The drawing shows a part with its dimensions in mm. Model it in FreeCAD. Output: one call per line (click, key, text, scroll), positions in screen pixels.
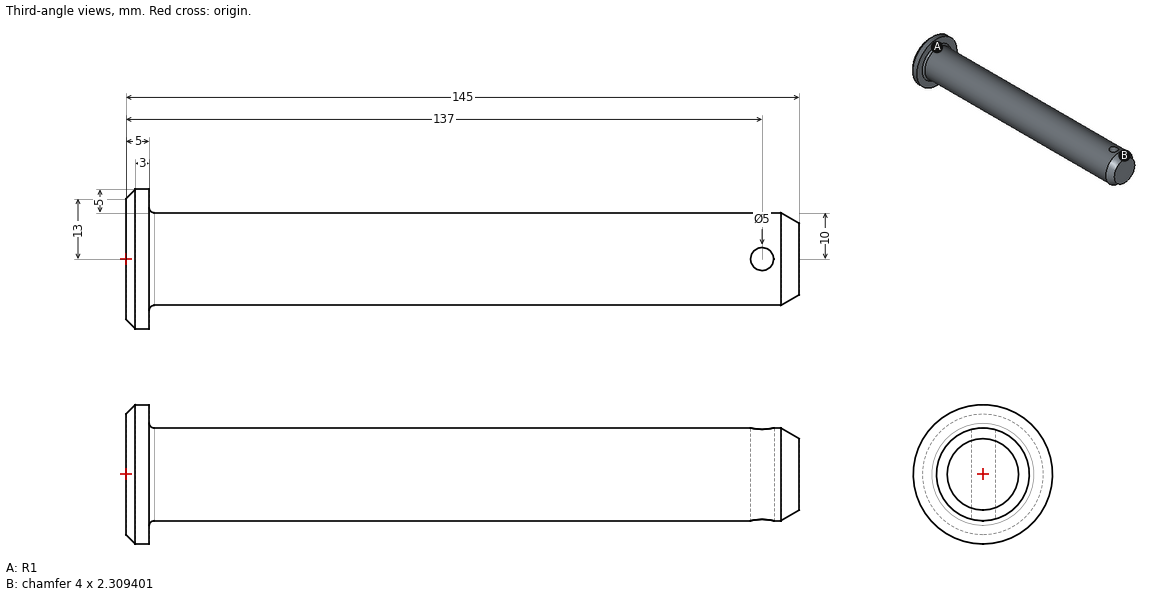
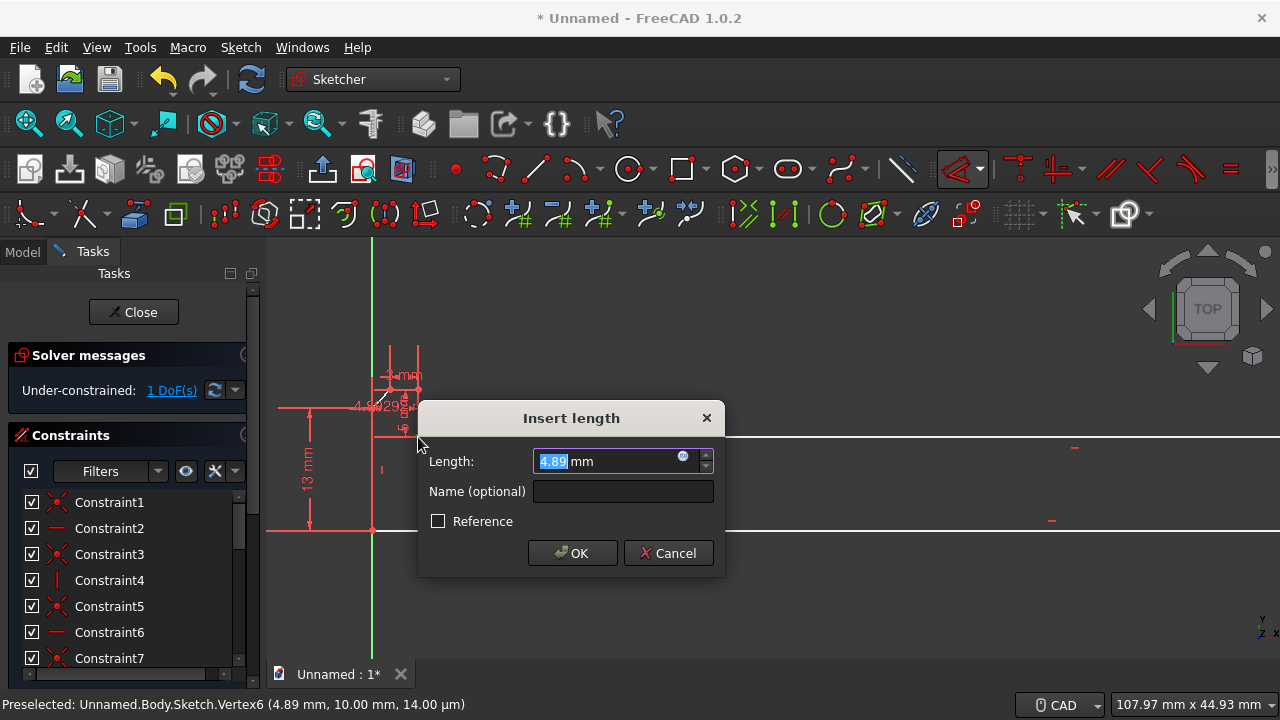
text(5)
key(Return)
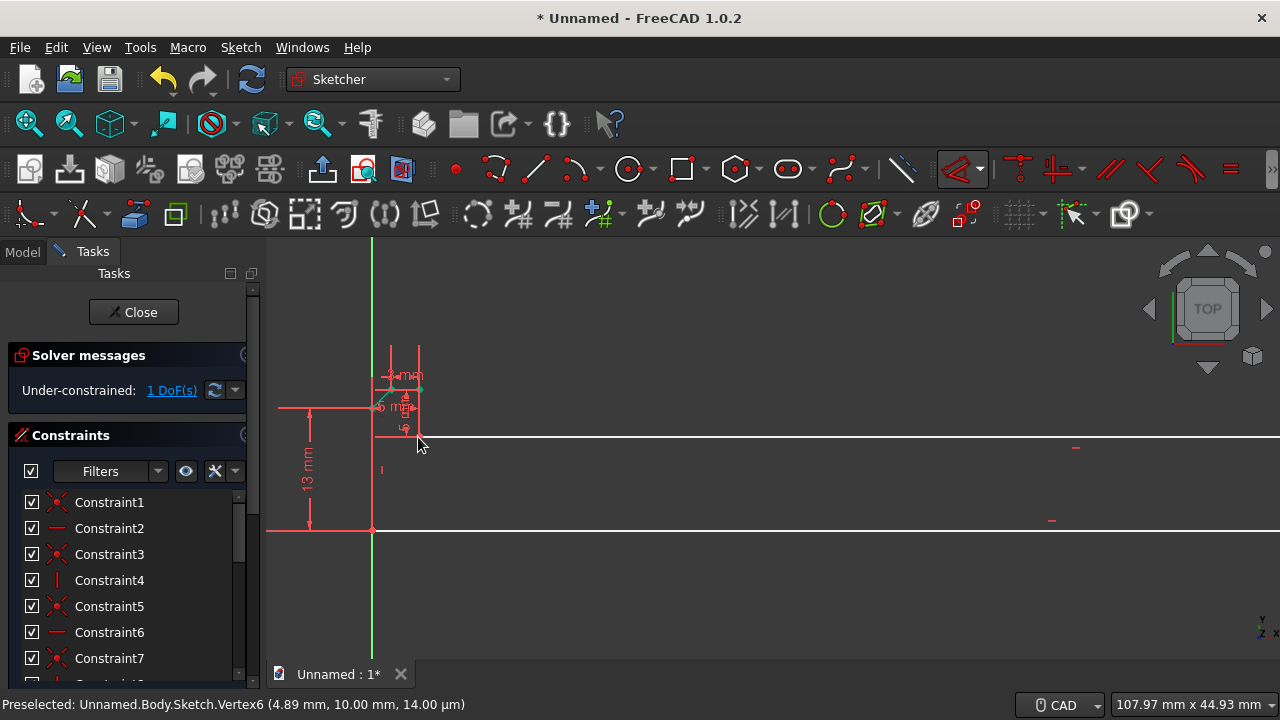
click(781, 531)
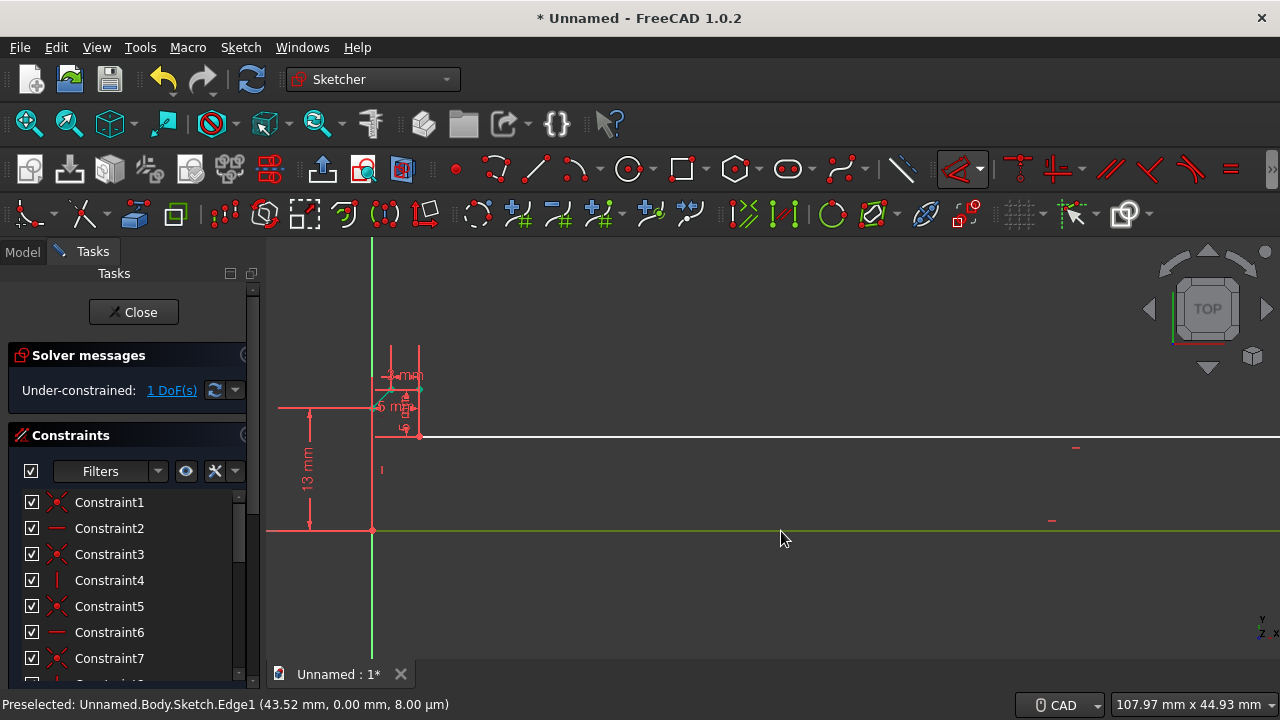
click(982, 170)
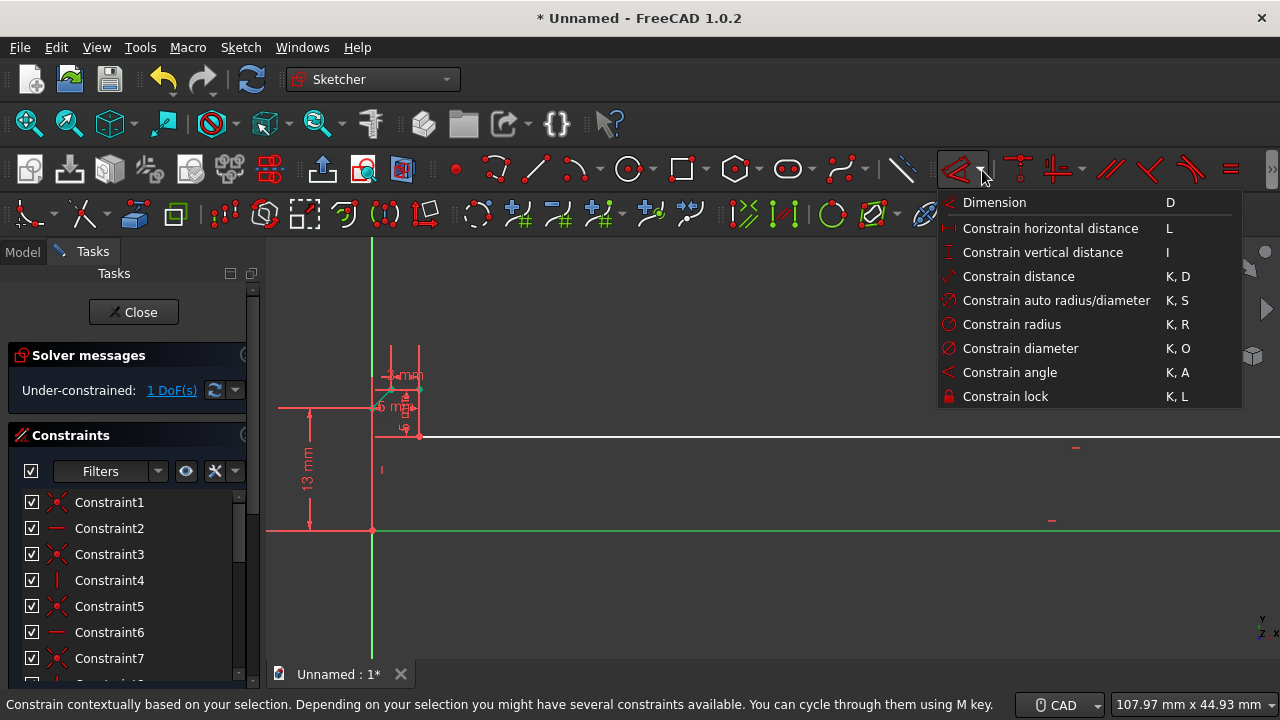
click(1090, 228)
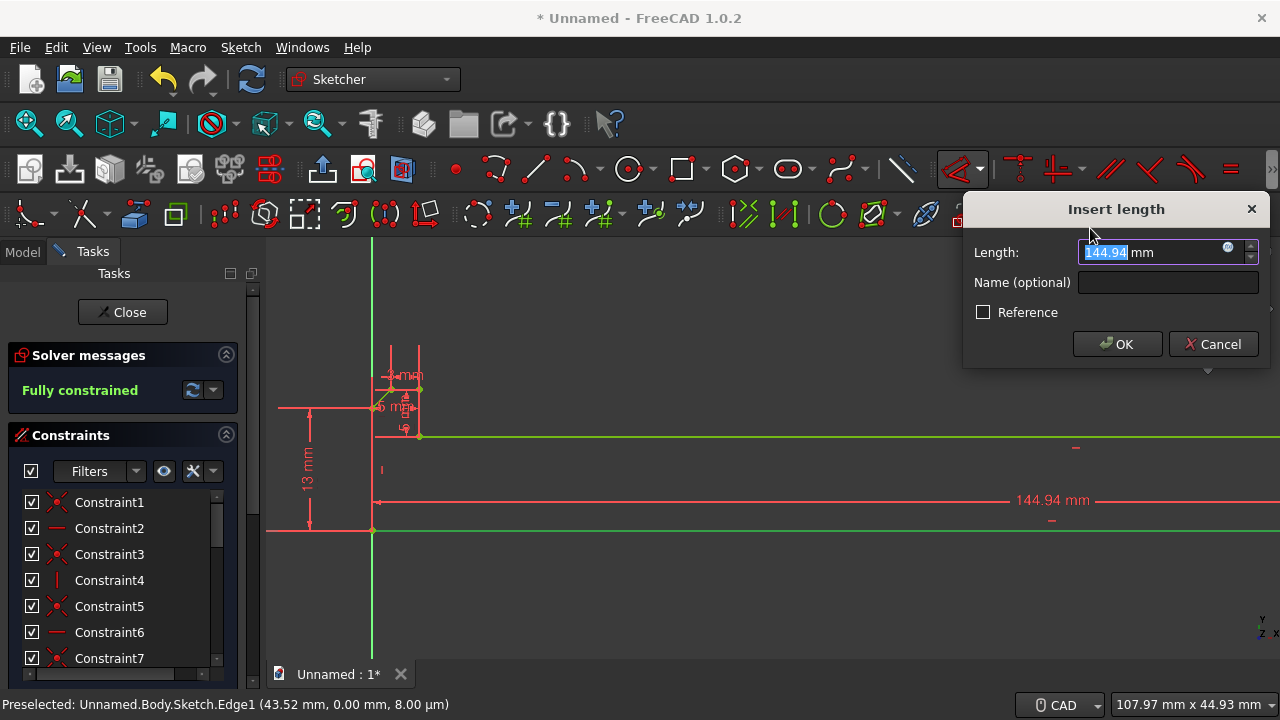
text(145)
key(Return)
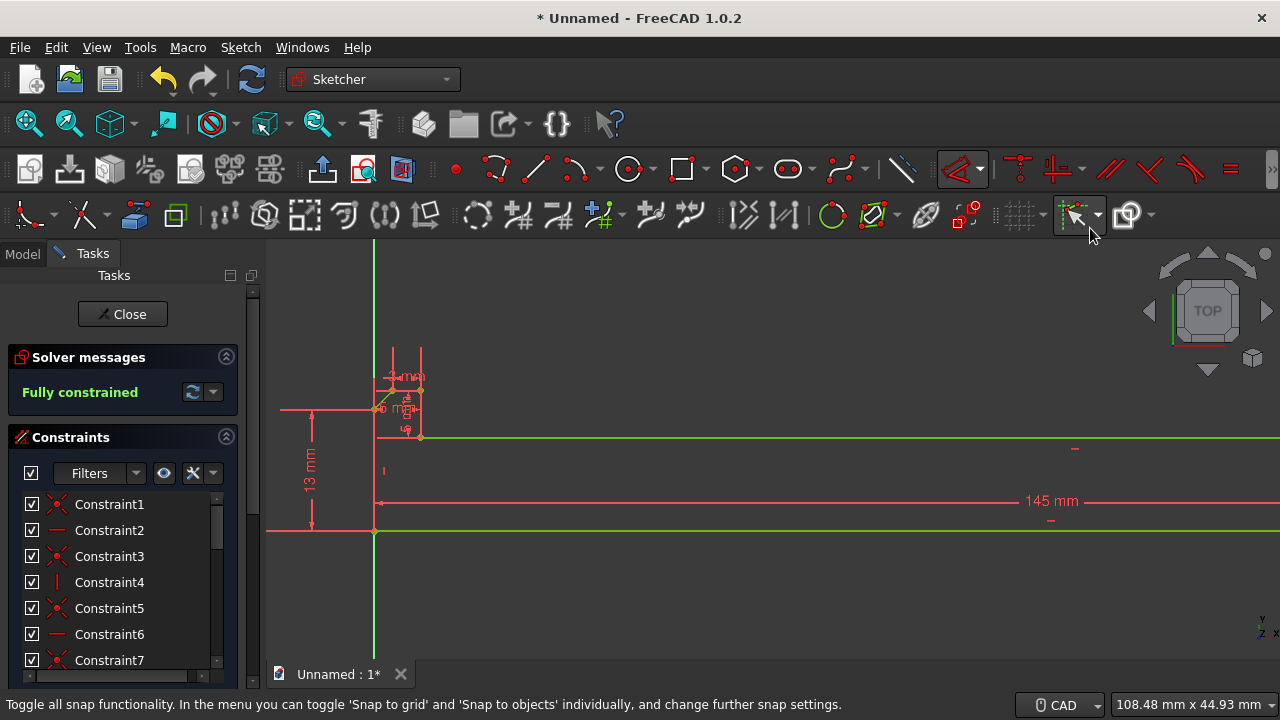
click(123, 314)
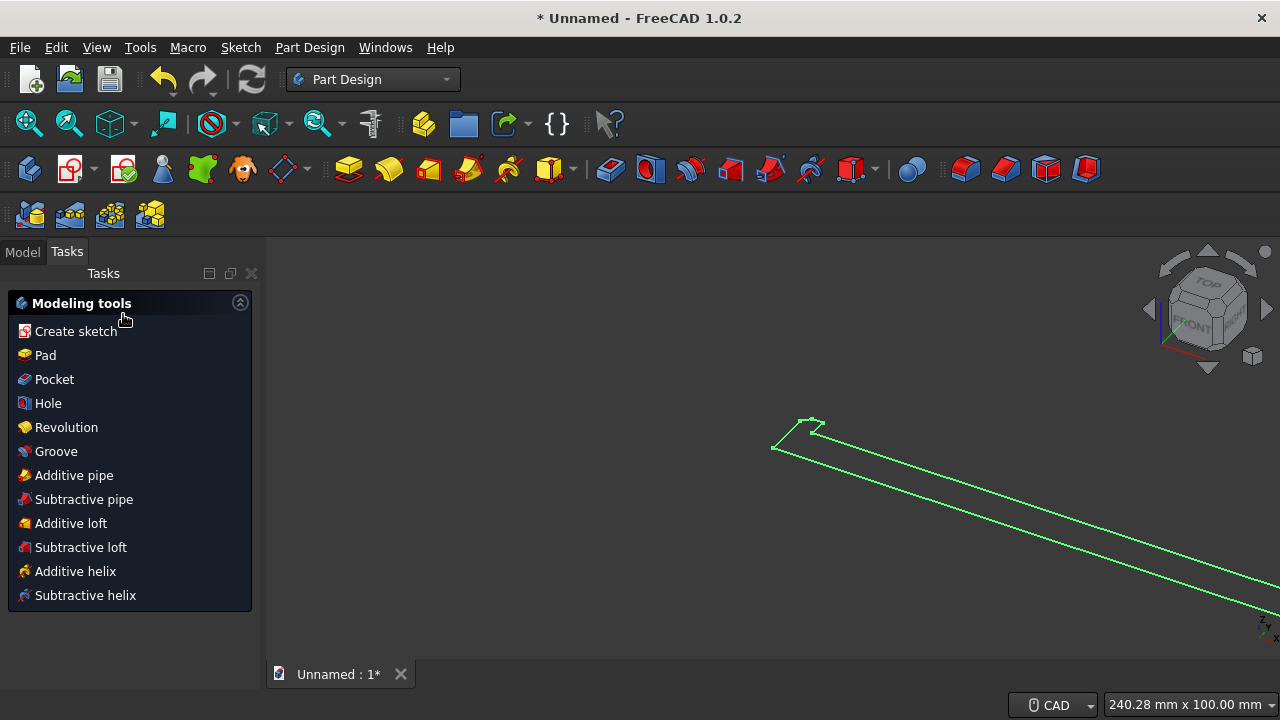
click(390, 170)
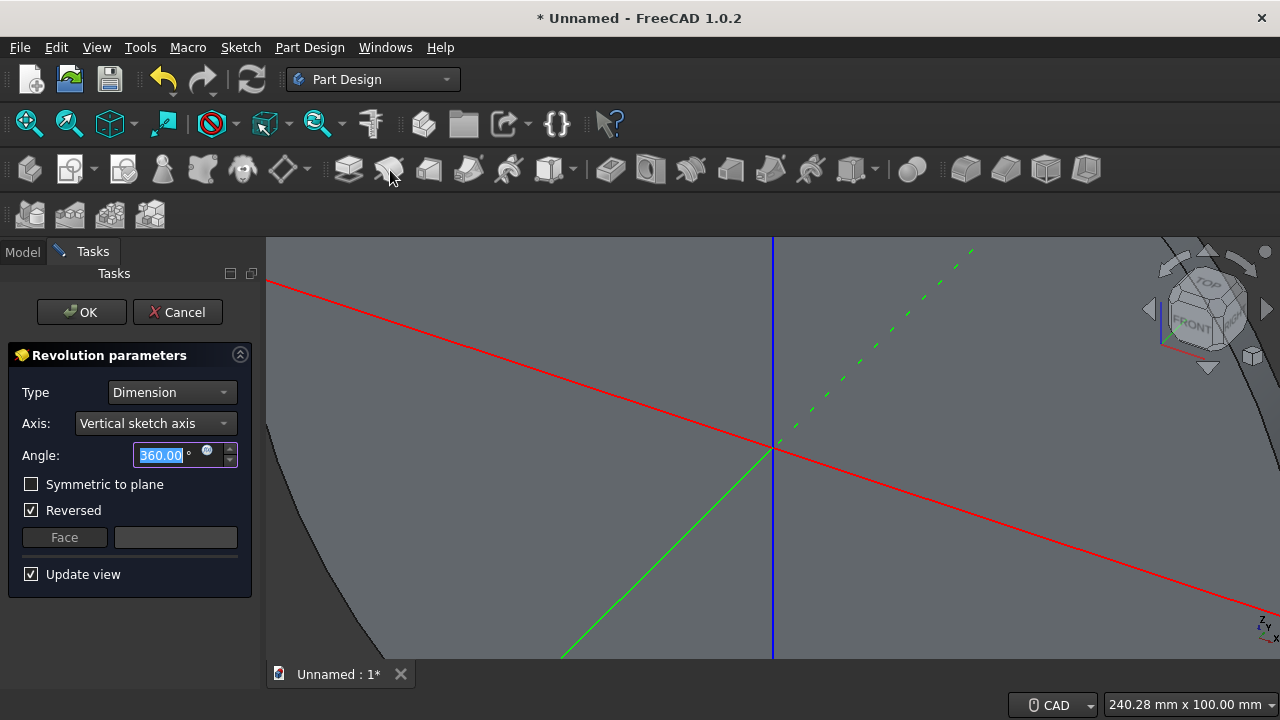
click(156, 424)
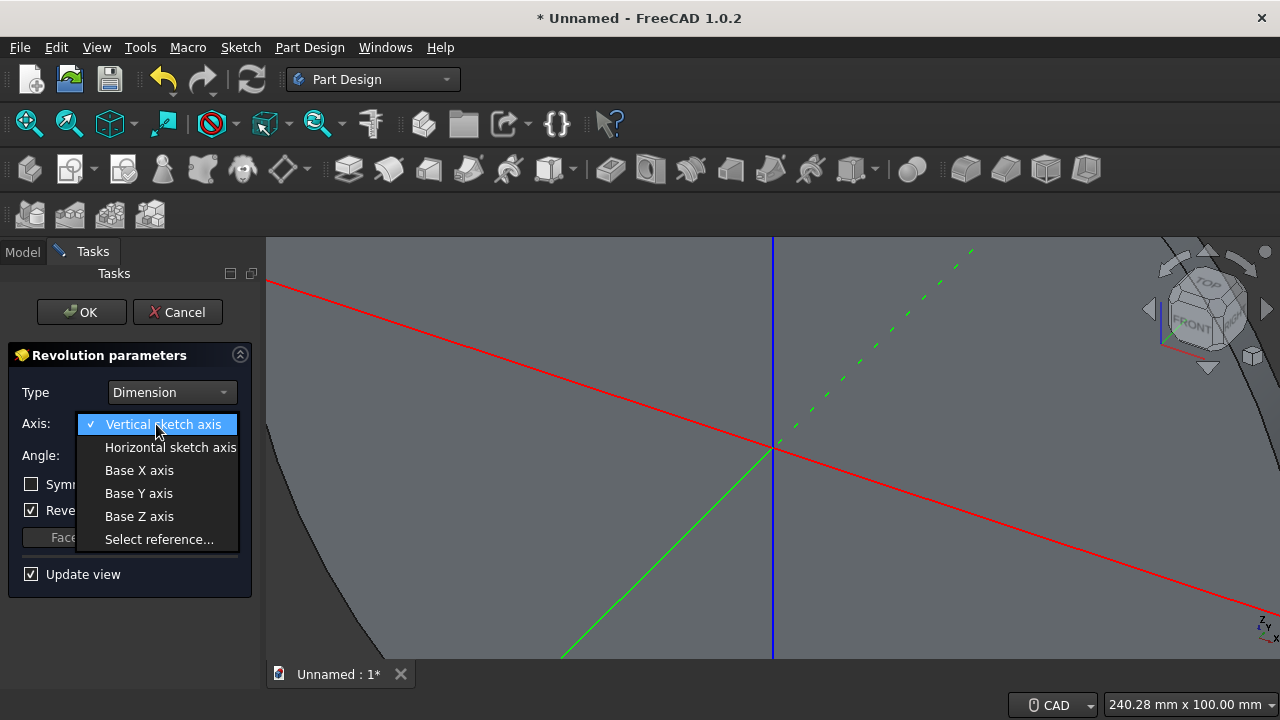
click(156, 448)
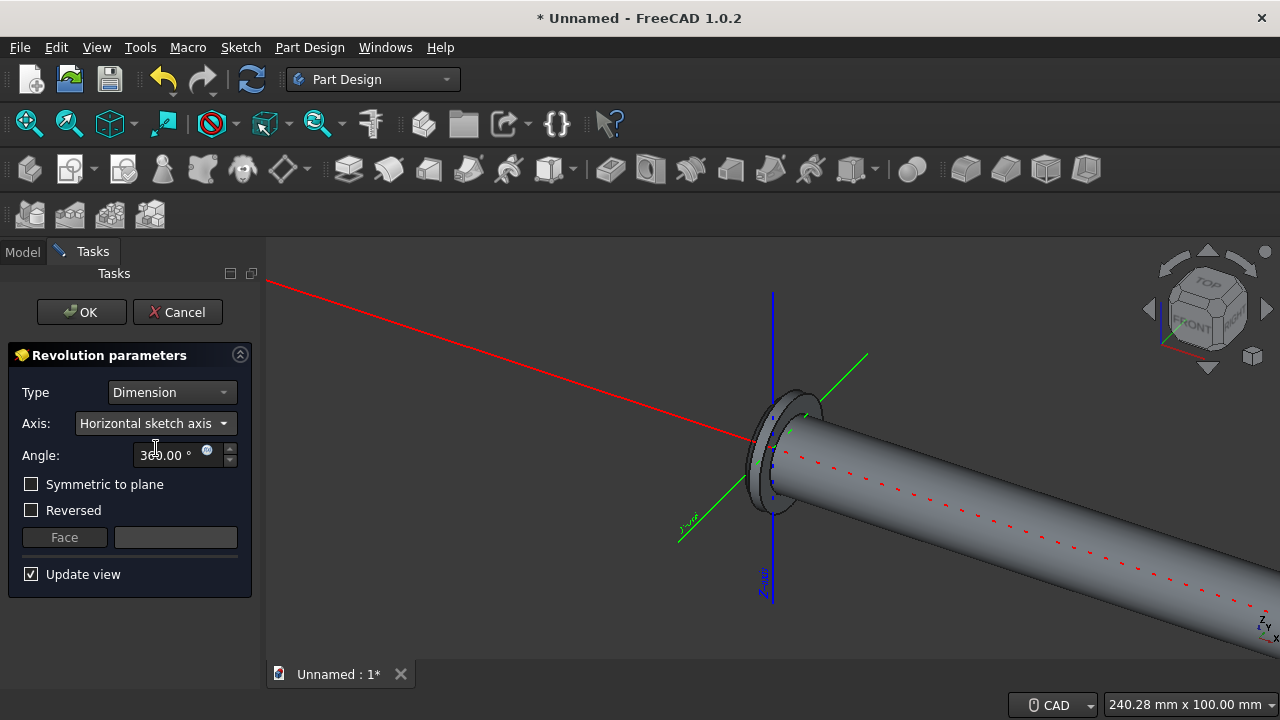
click(82, 312)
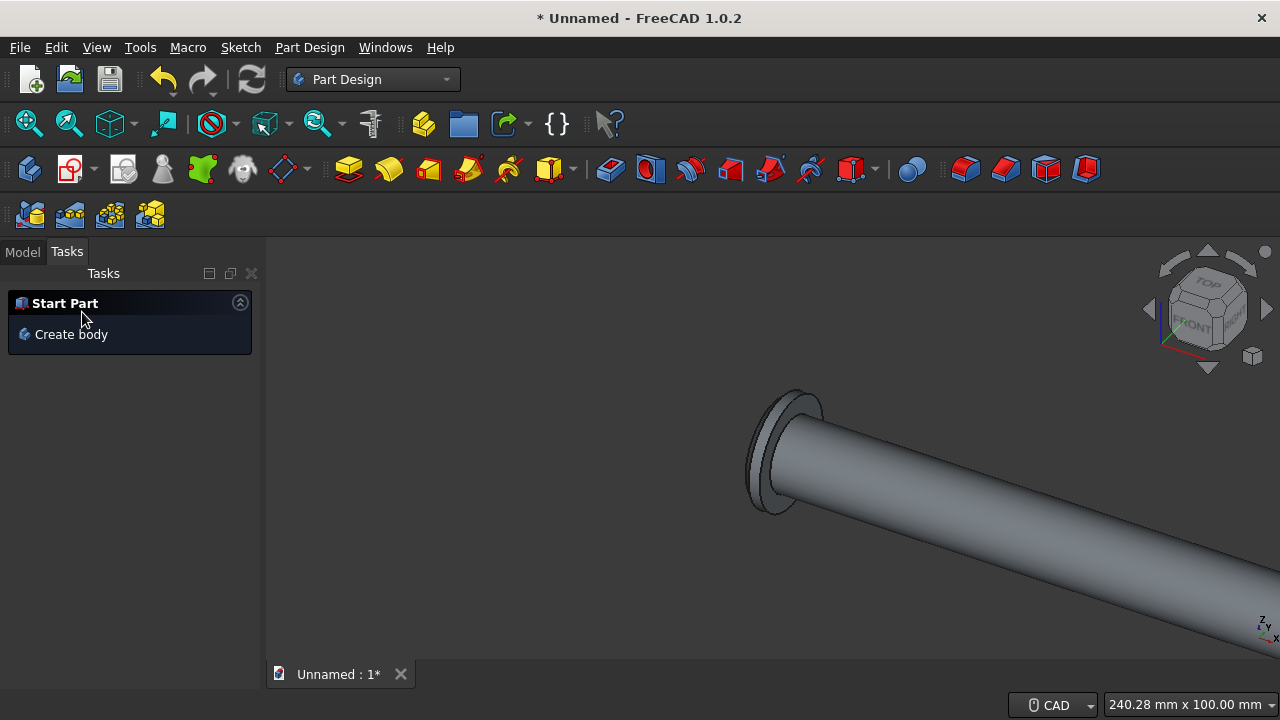
key(v)
key(f)